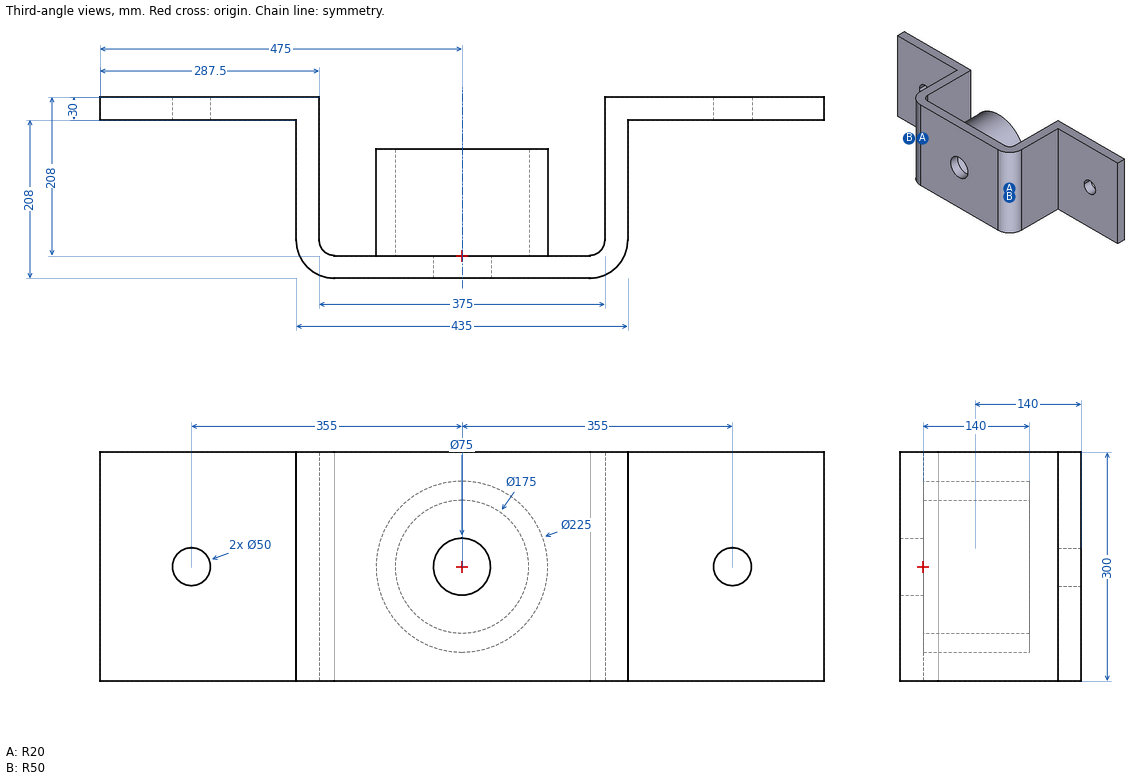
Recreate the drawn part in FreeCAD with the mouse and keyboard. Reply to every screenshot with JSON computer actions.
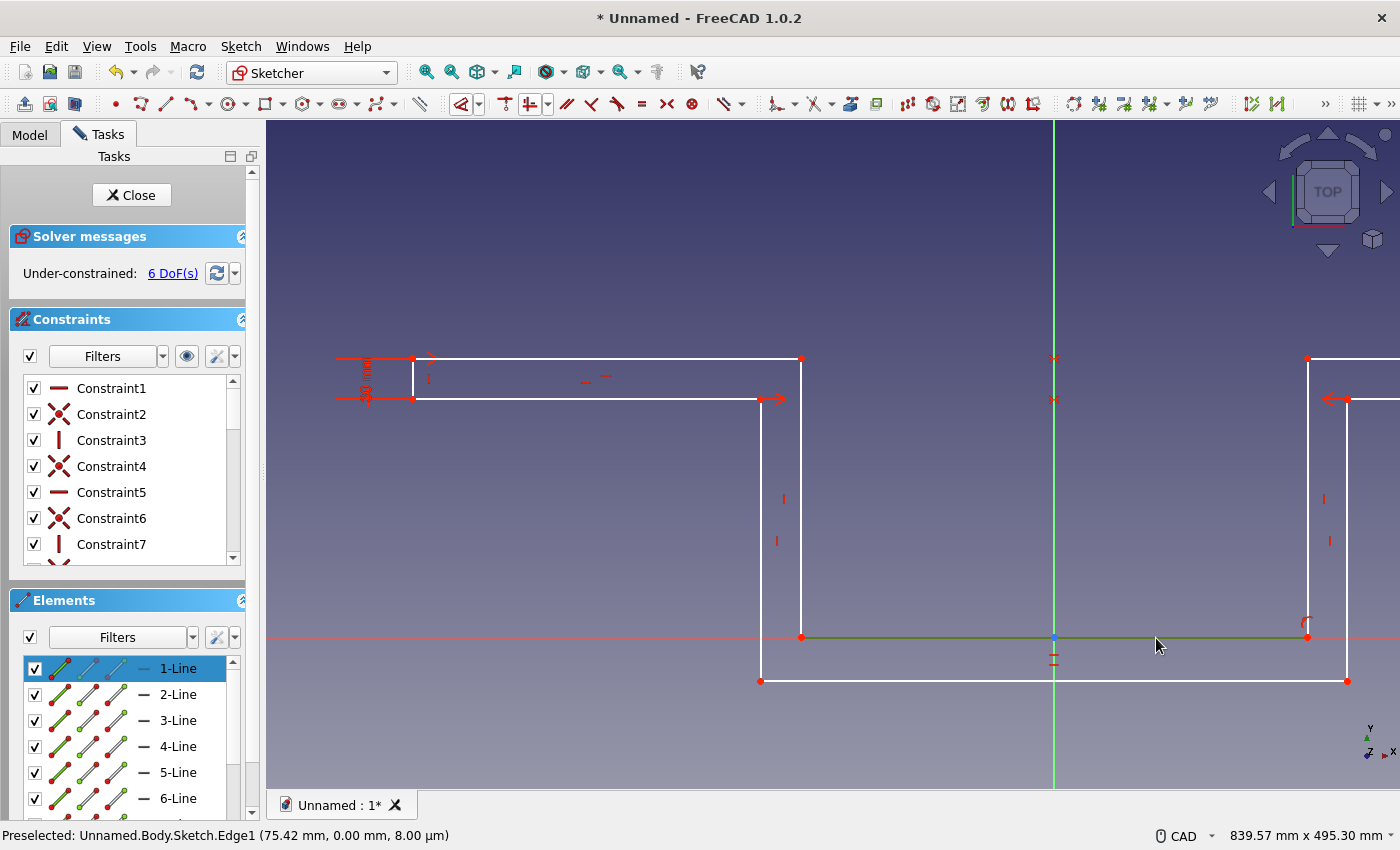
{"action": "left_click", "coordinate": [478, 104]}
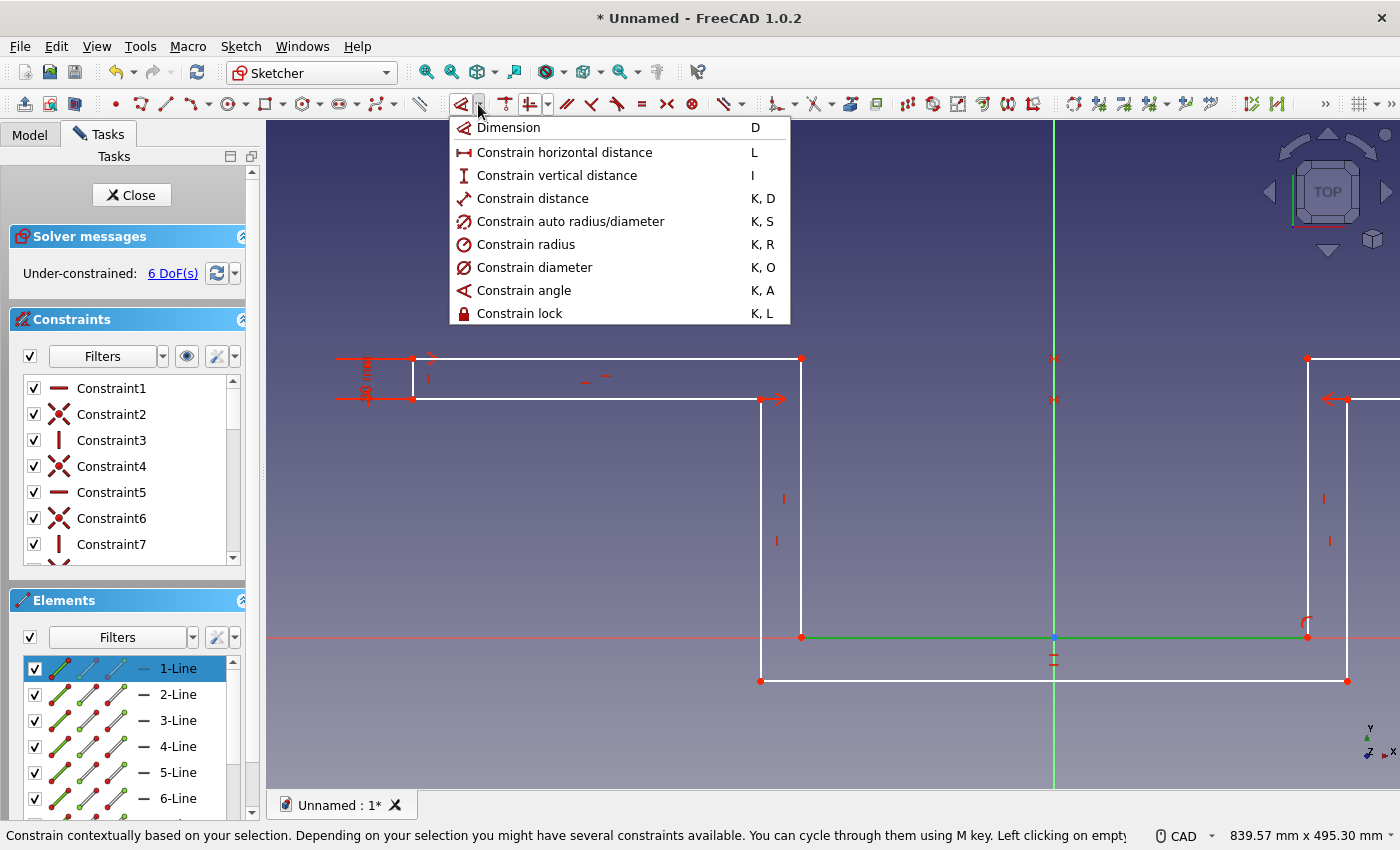
{"action": "left_click", "coordinate": [620, 152]}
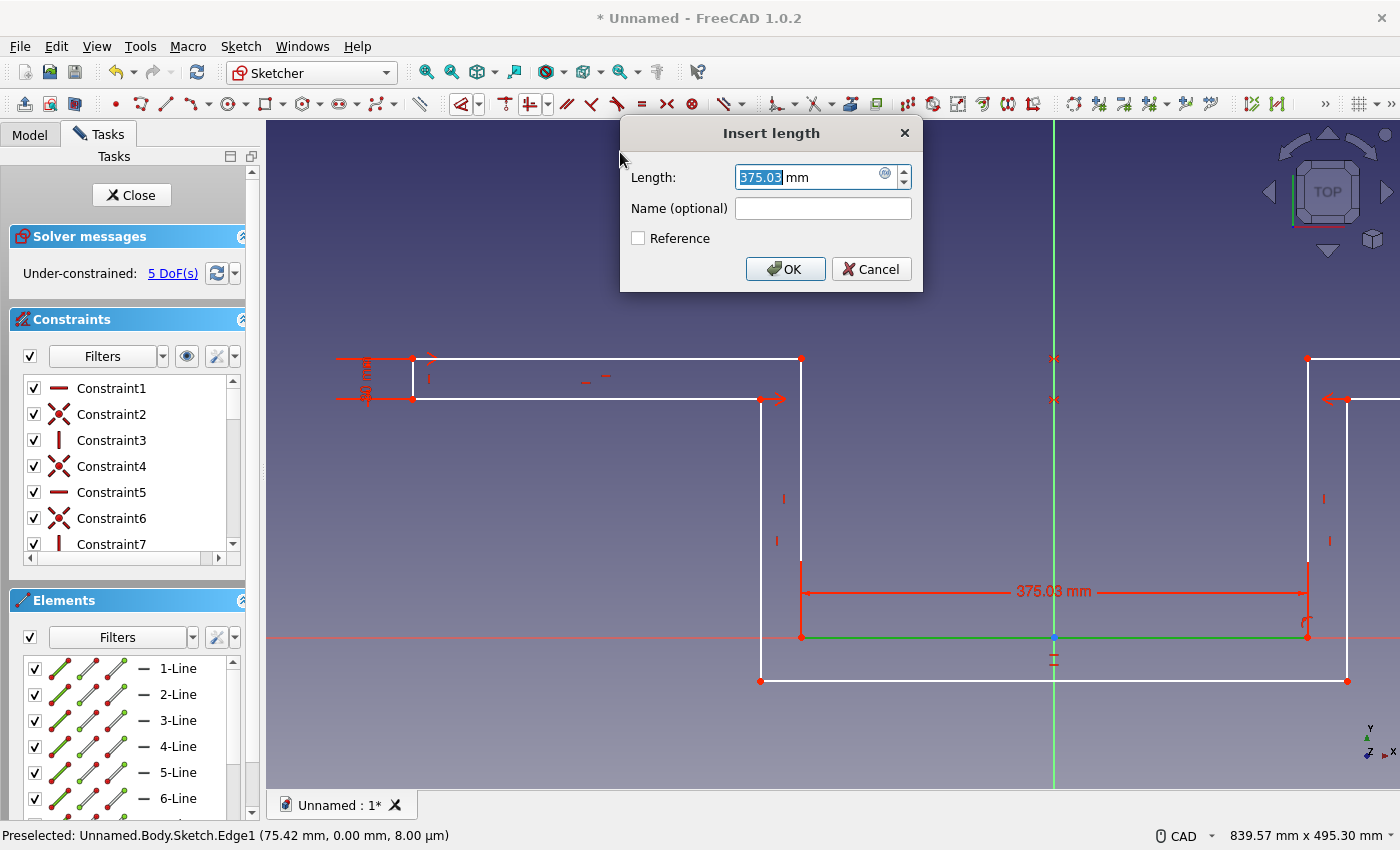
{"action": "type", "text": "375"}
{"action": "key", "text": "Return"}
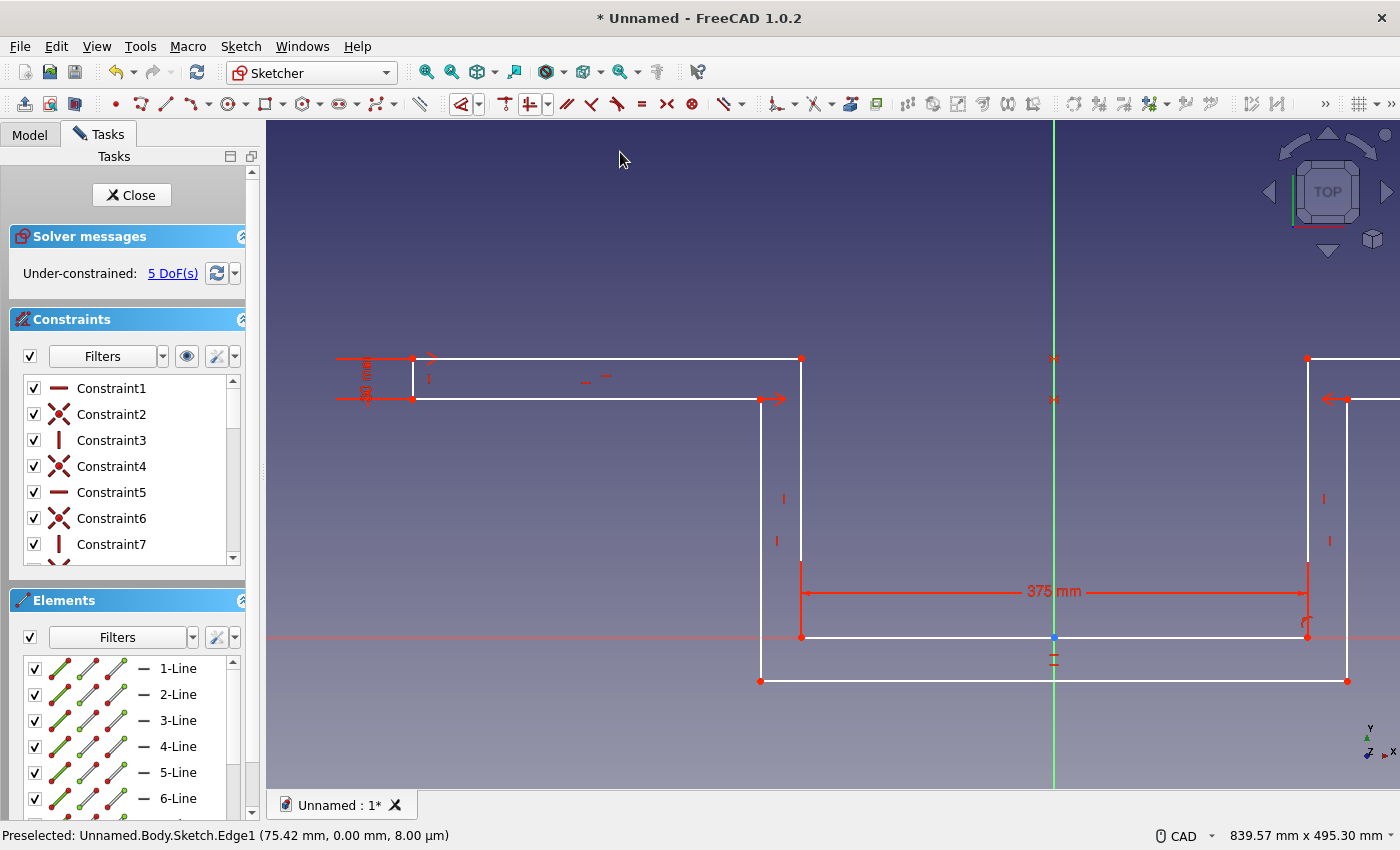
{"action": "left_click", "coordinate": [801, 554]}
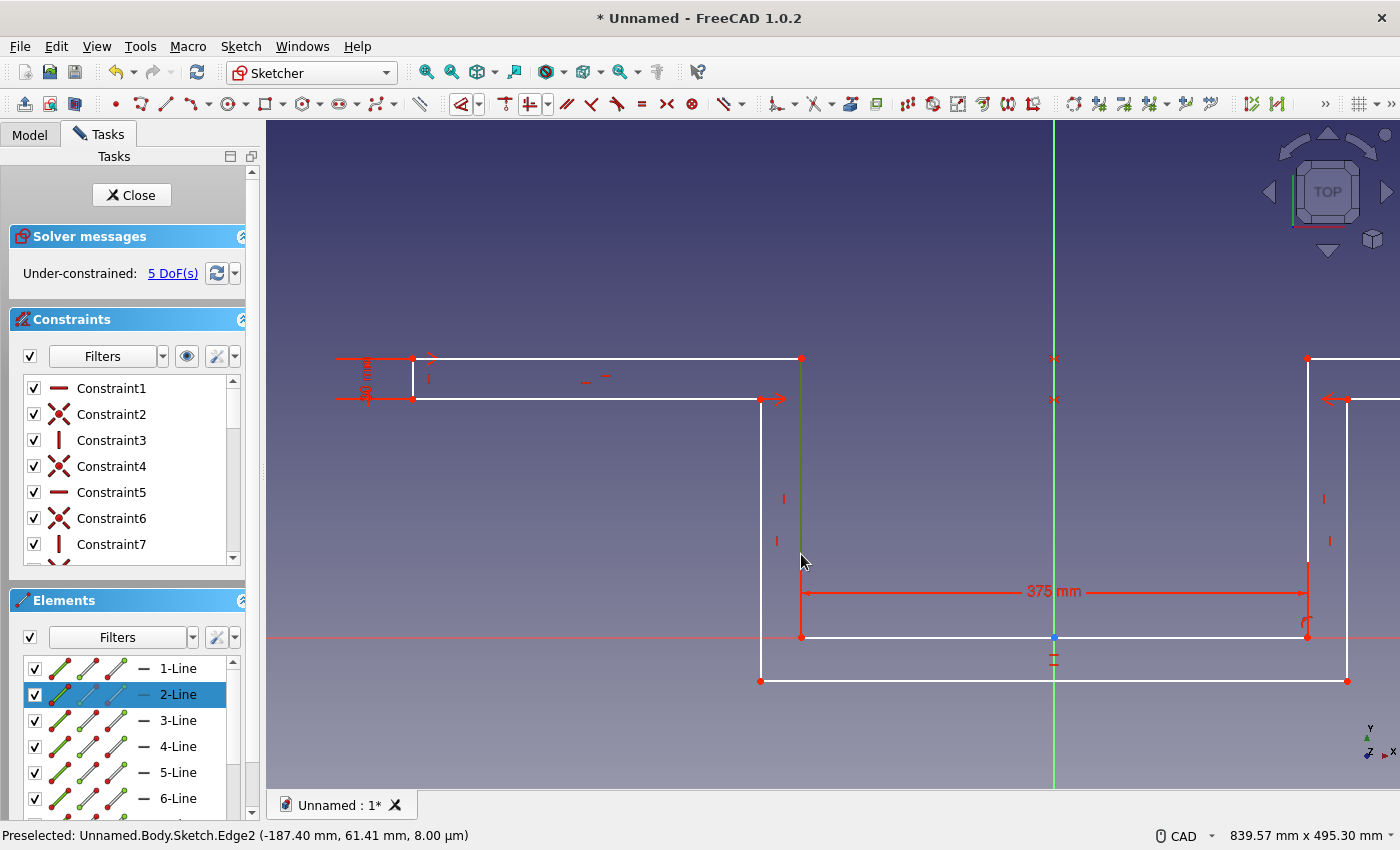
{"action": "left_click", "coordinate": [478, 104]}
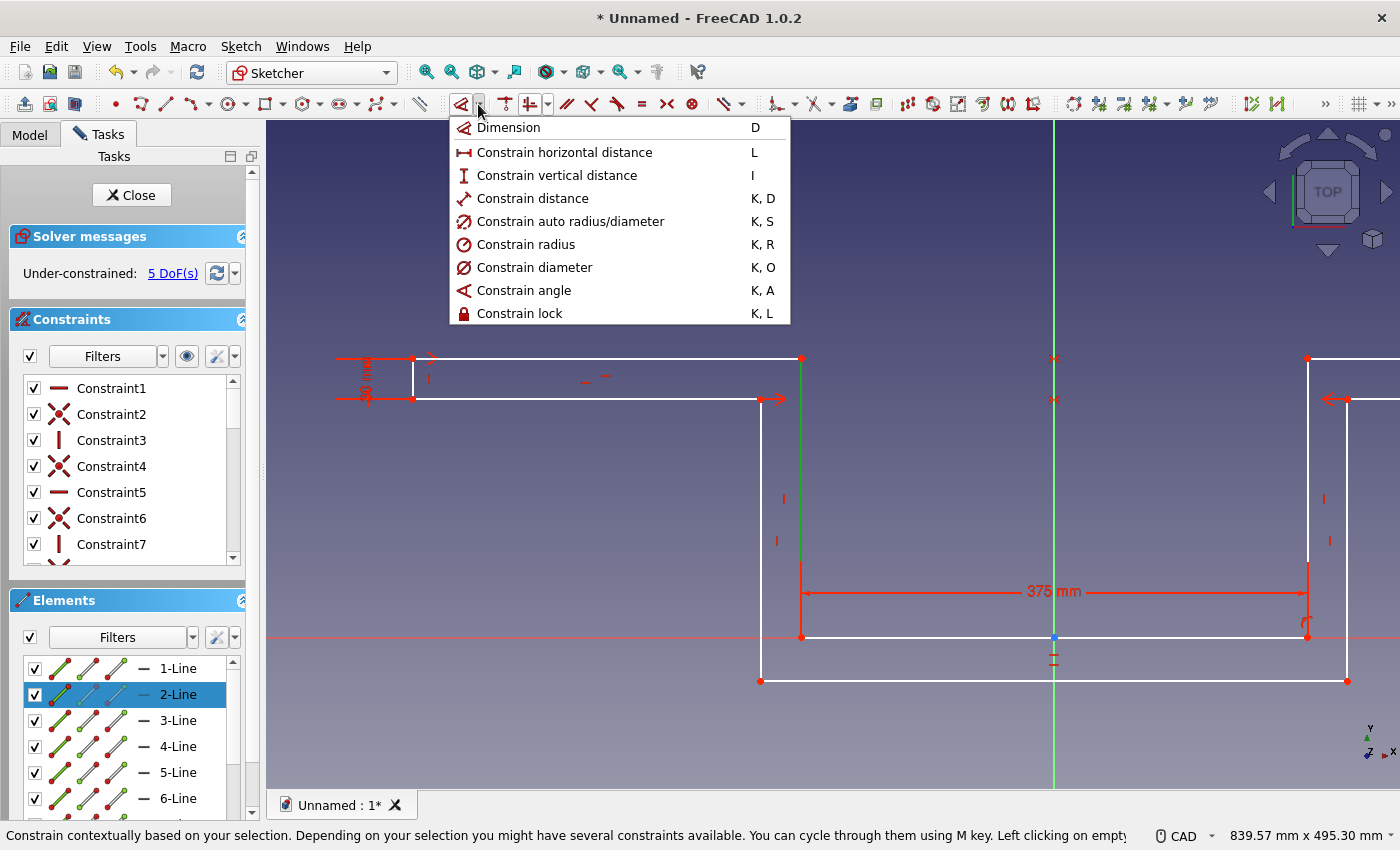
{"action": "left_click", "coordinate": [620, 176]}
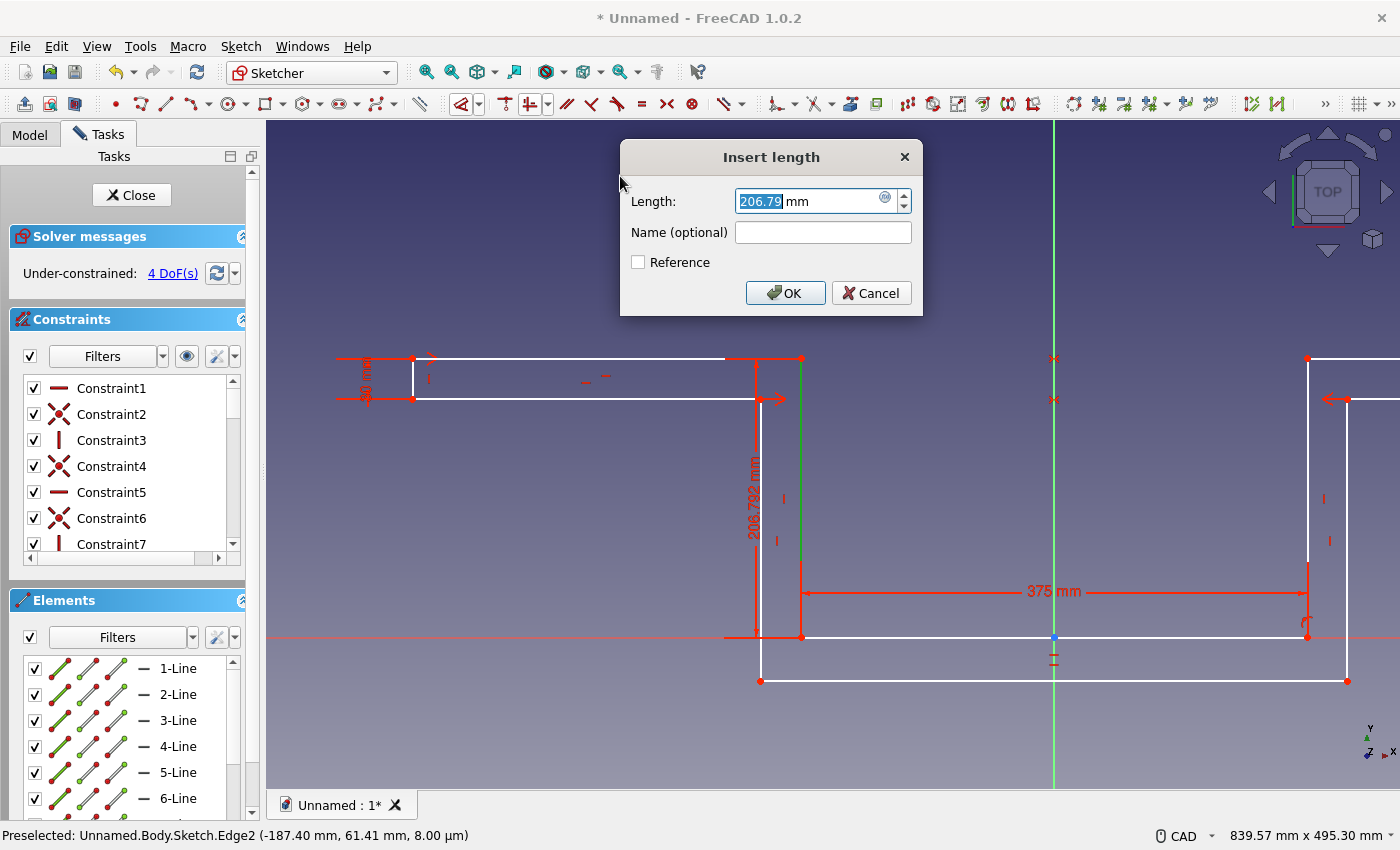
{"action": "type", "text": "208"}
{"action": "key", "text": "Return"}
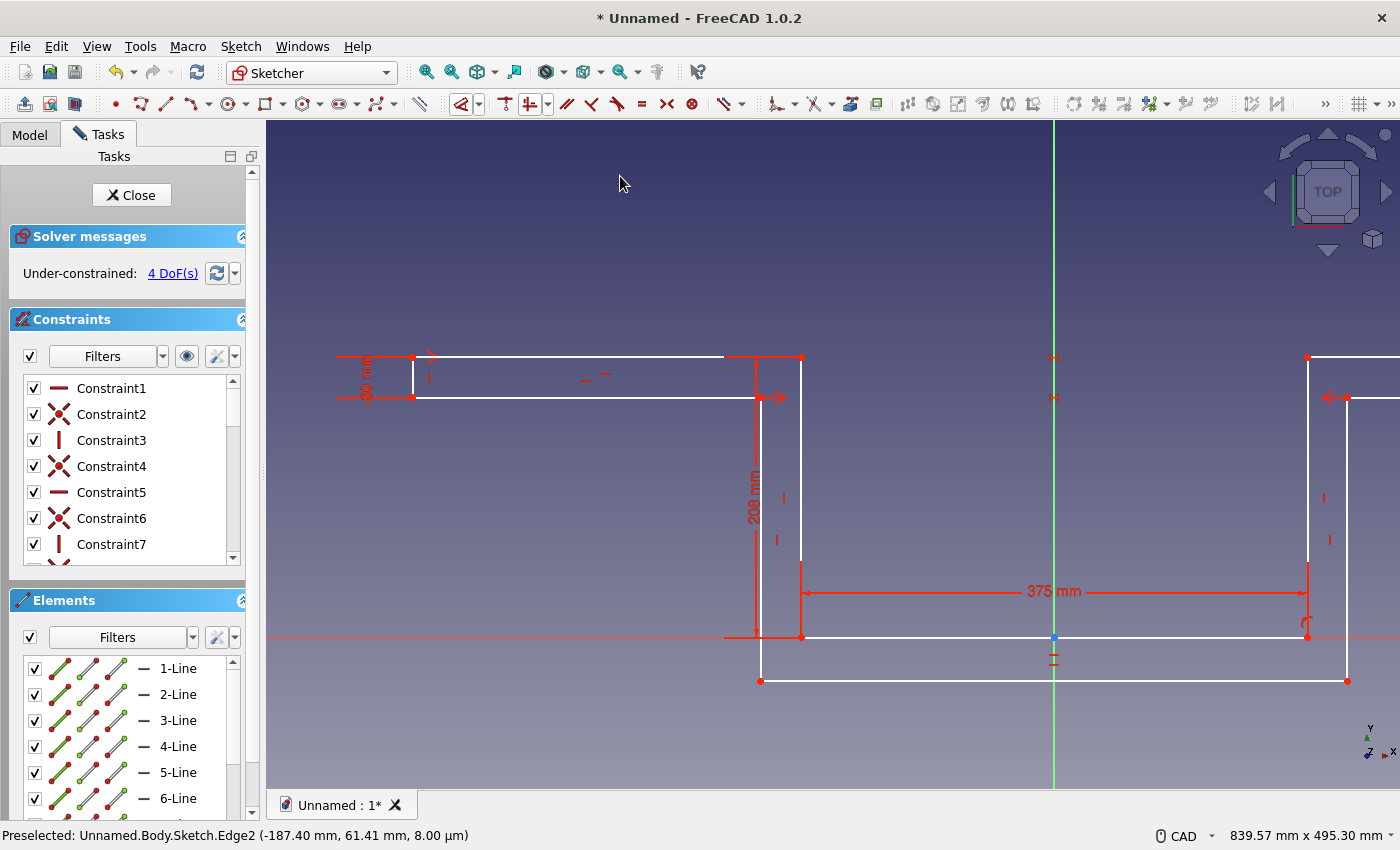
{"action": "left_click", "coordinate": [761, 596]}